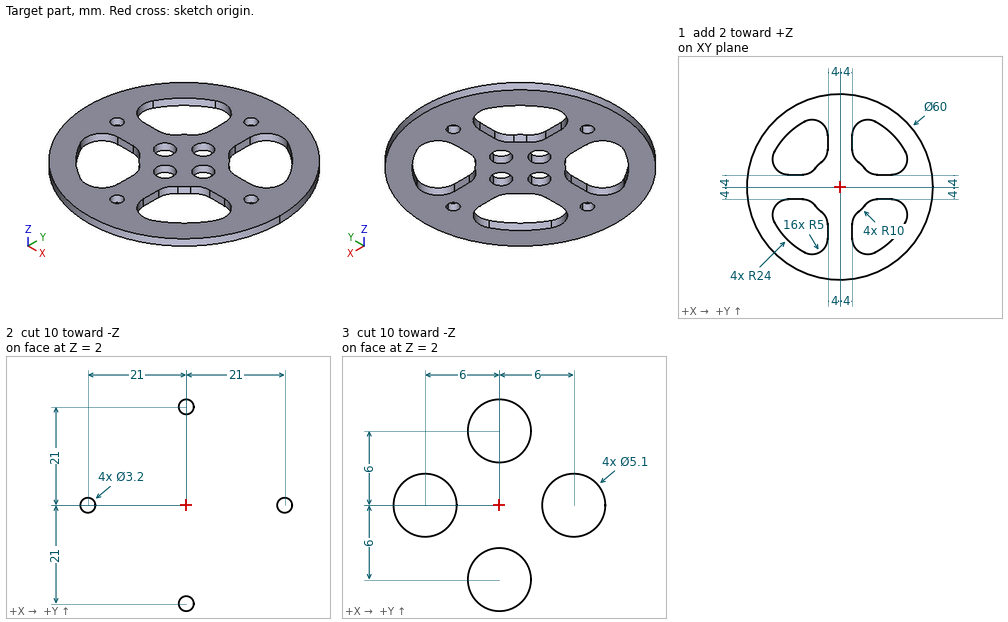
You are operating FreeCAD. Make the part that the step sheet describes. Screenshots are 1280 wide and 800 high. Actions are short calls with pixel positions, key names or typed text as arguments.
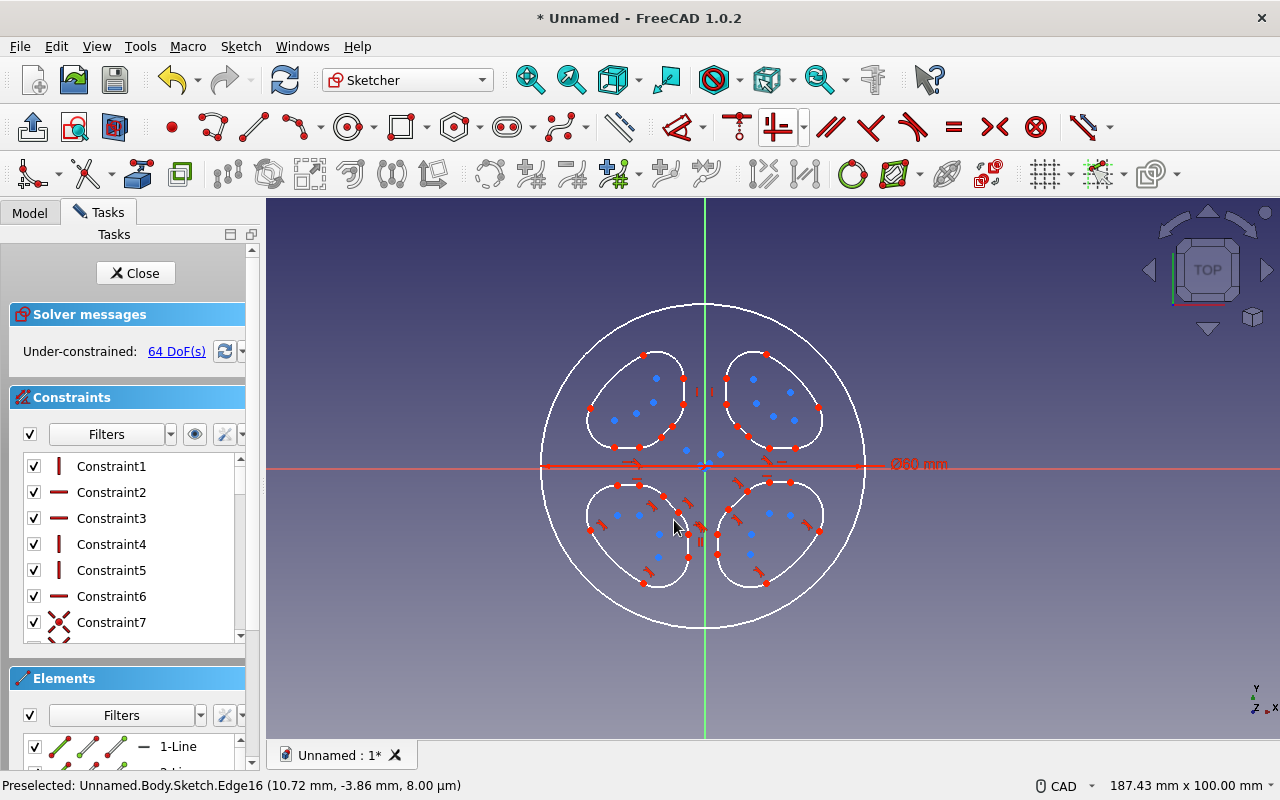
scroll(684, 387, up, 3)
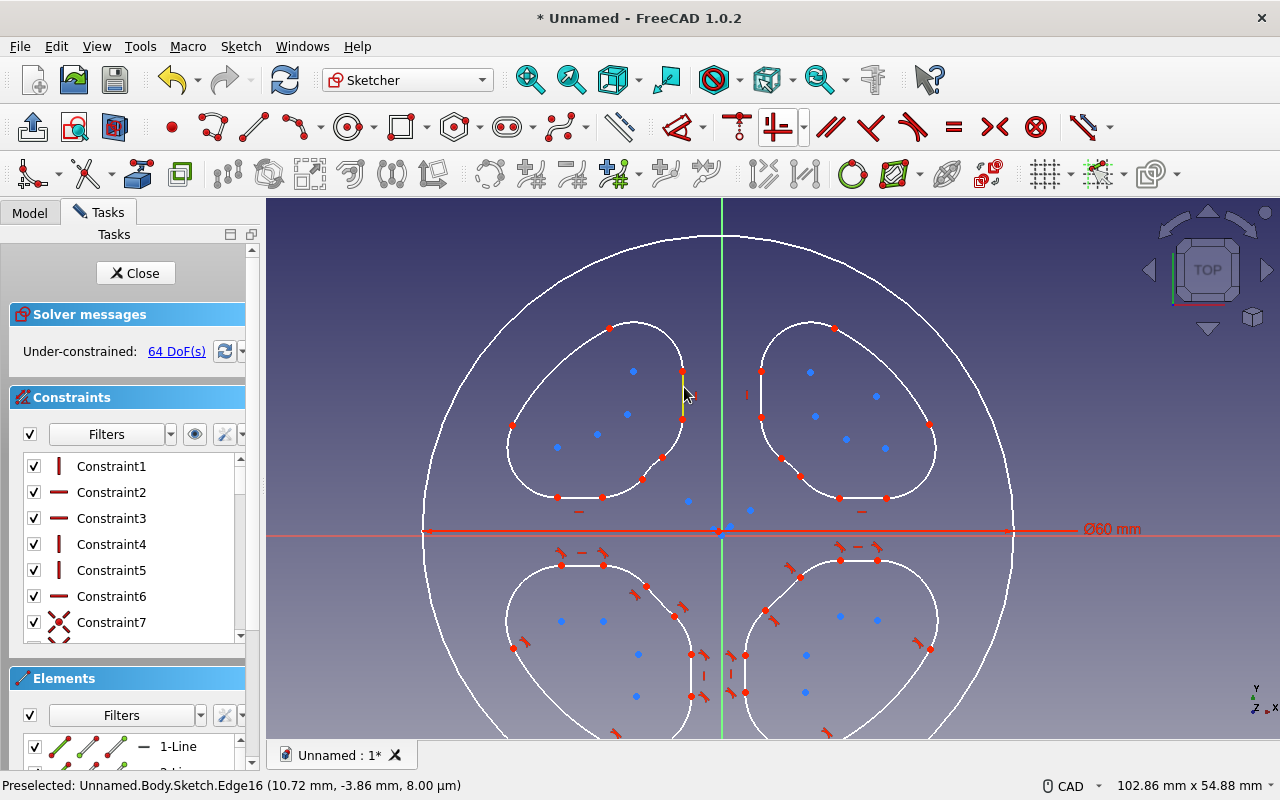
click(683, 386)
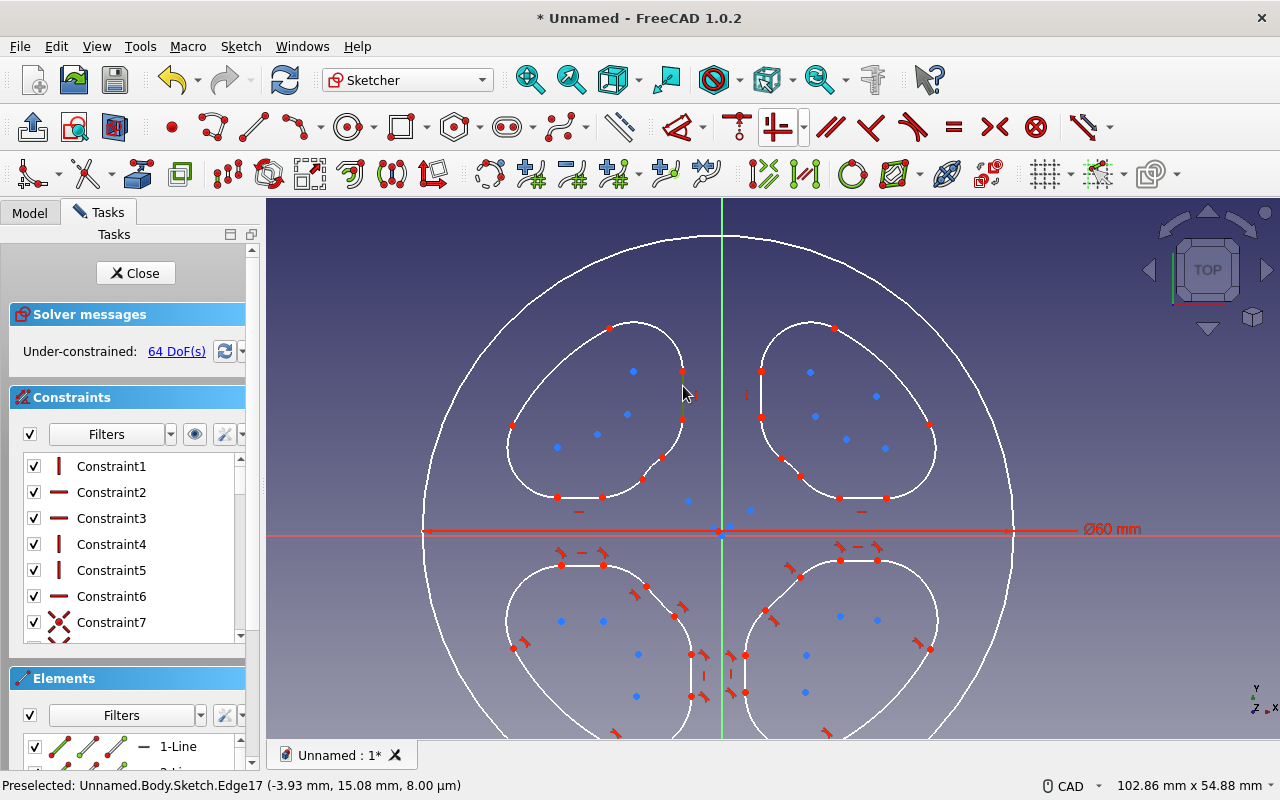
click(672, 448)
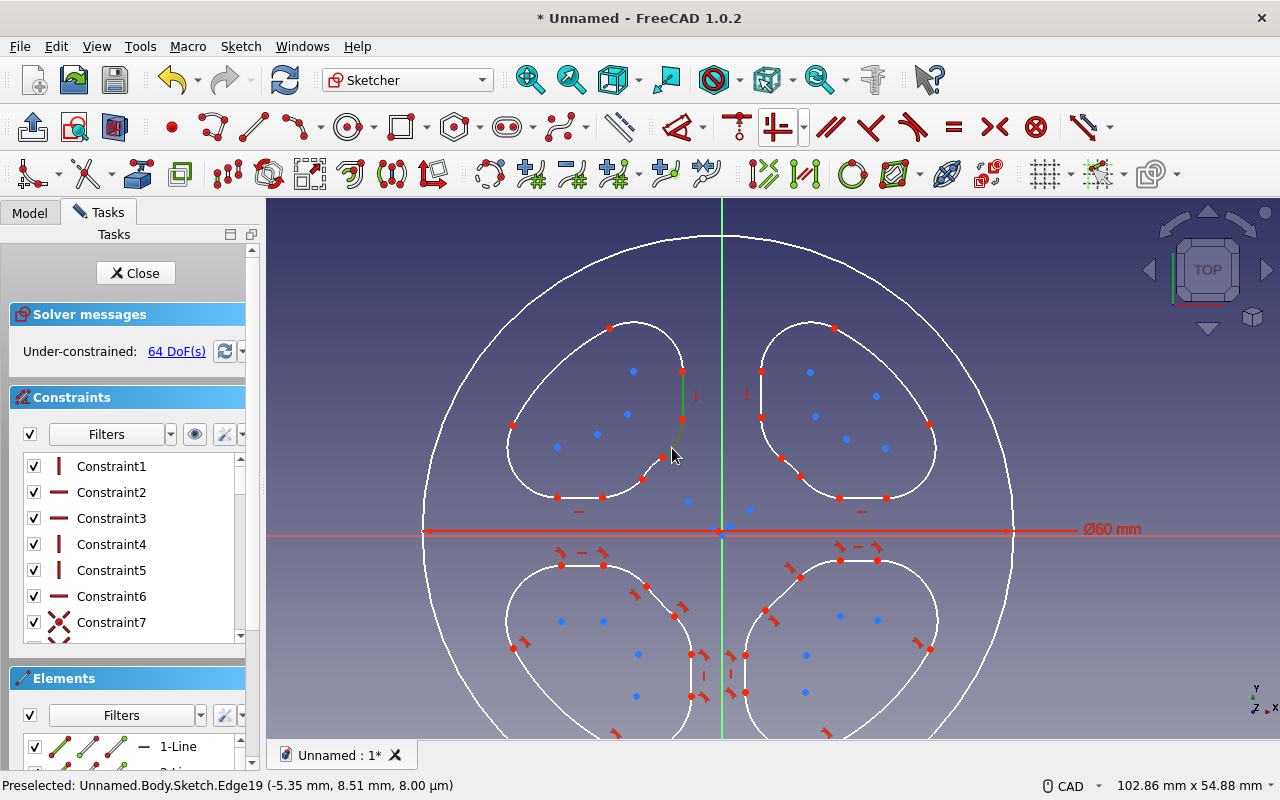
key(t)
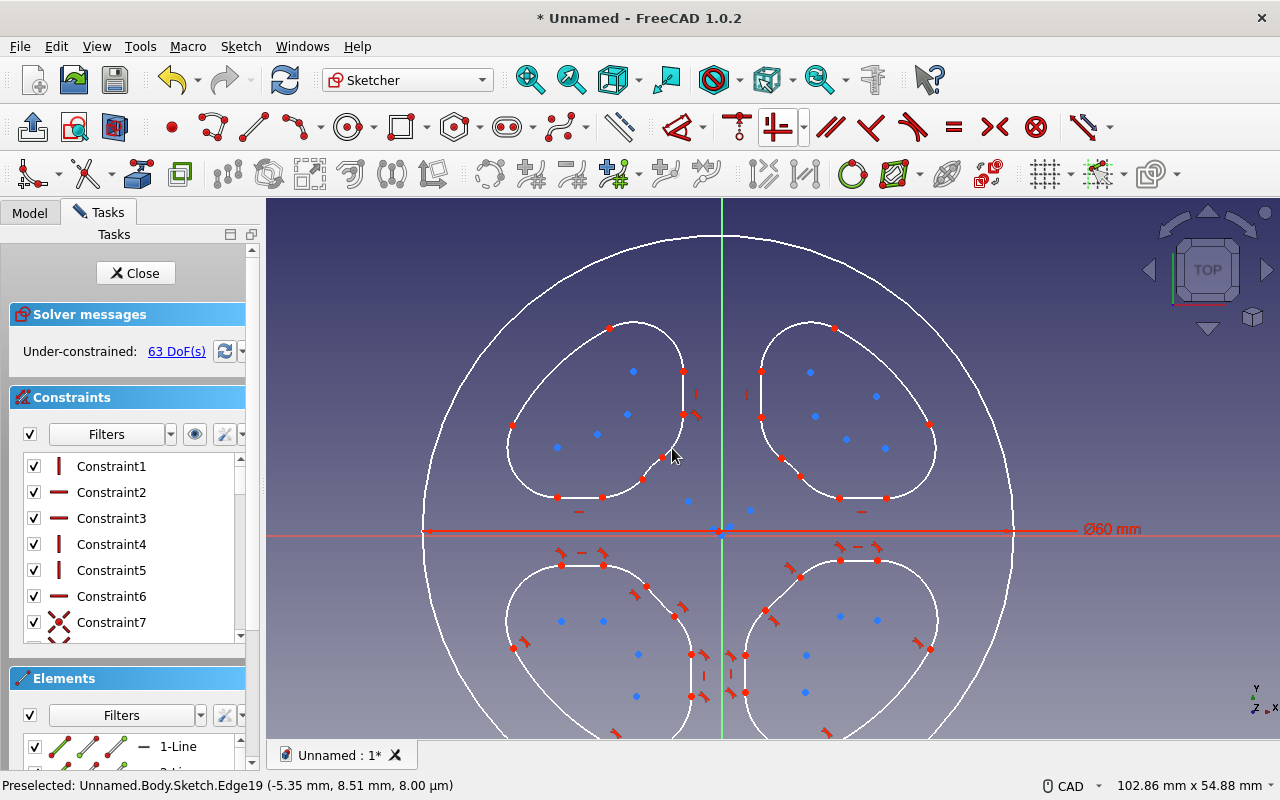
click(683, 385)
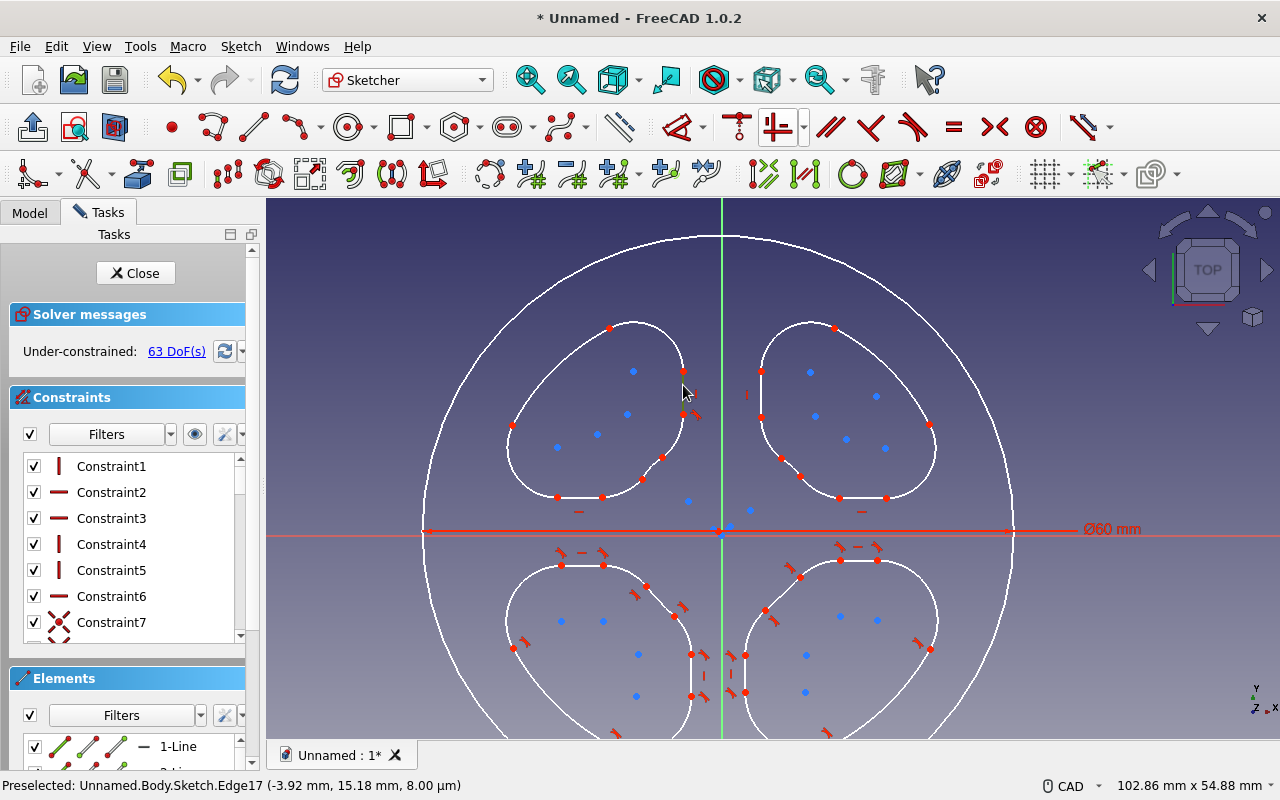
click(674, 343)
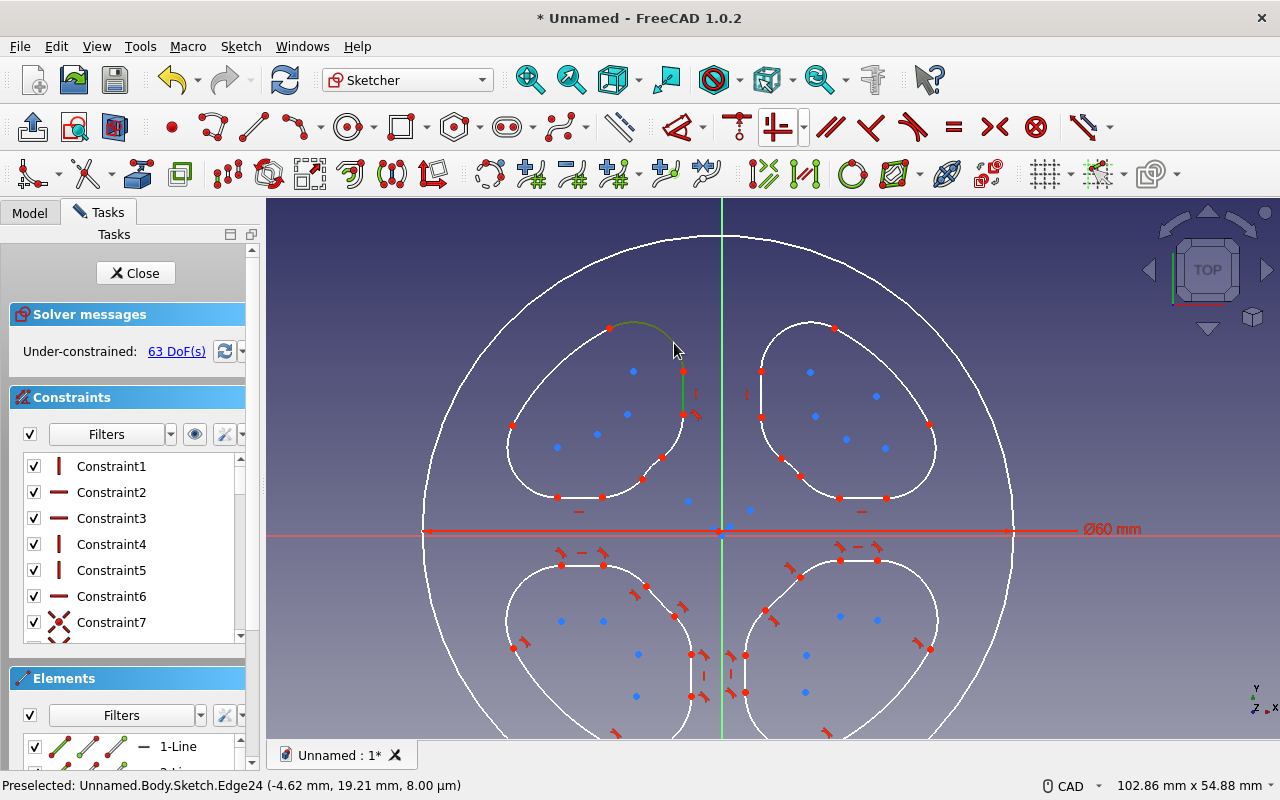
click(913, 128)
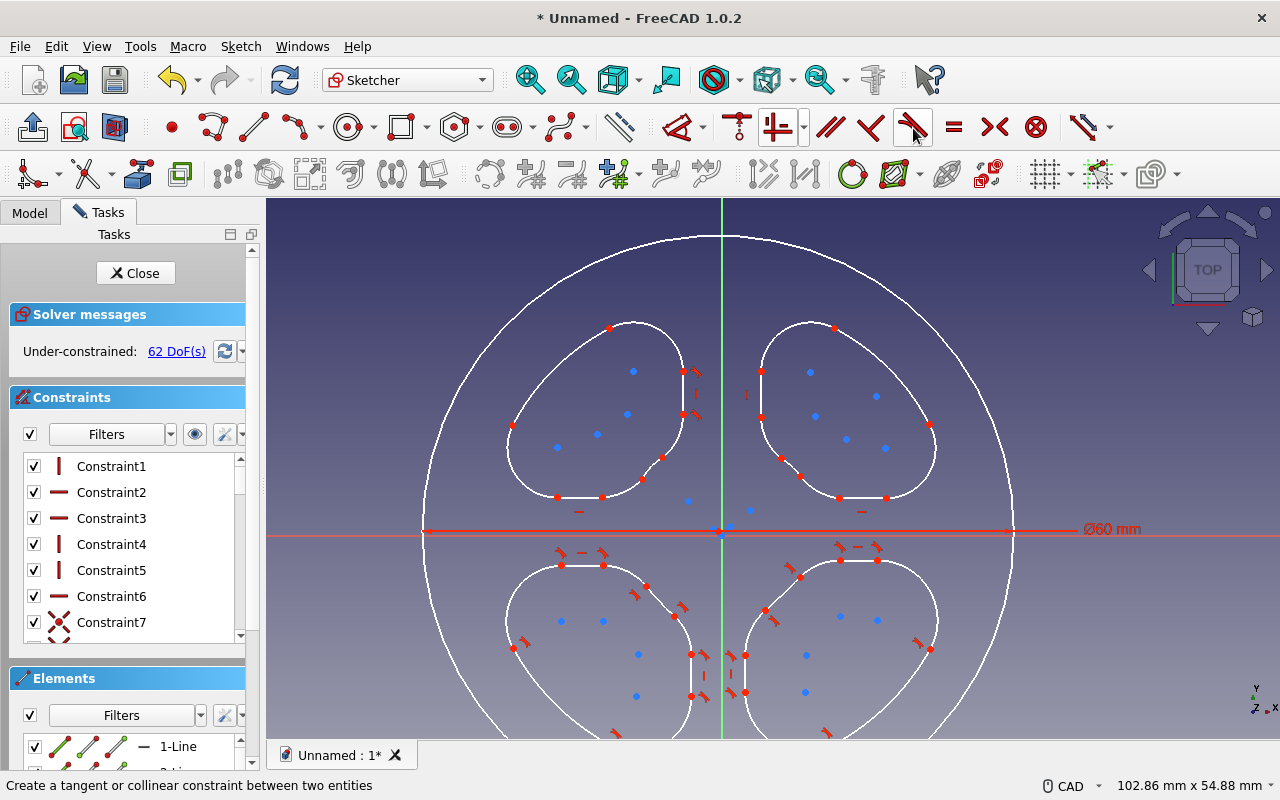
click(589, 498)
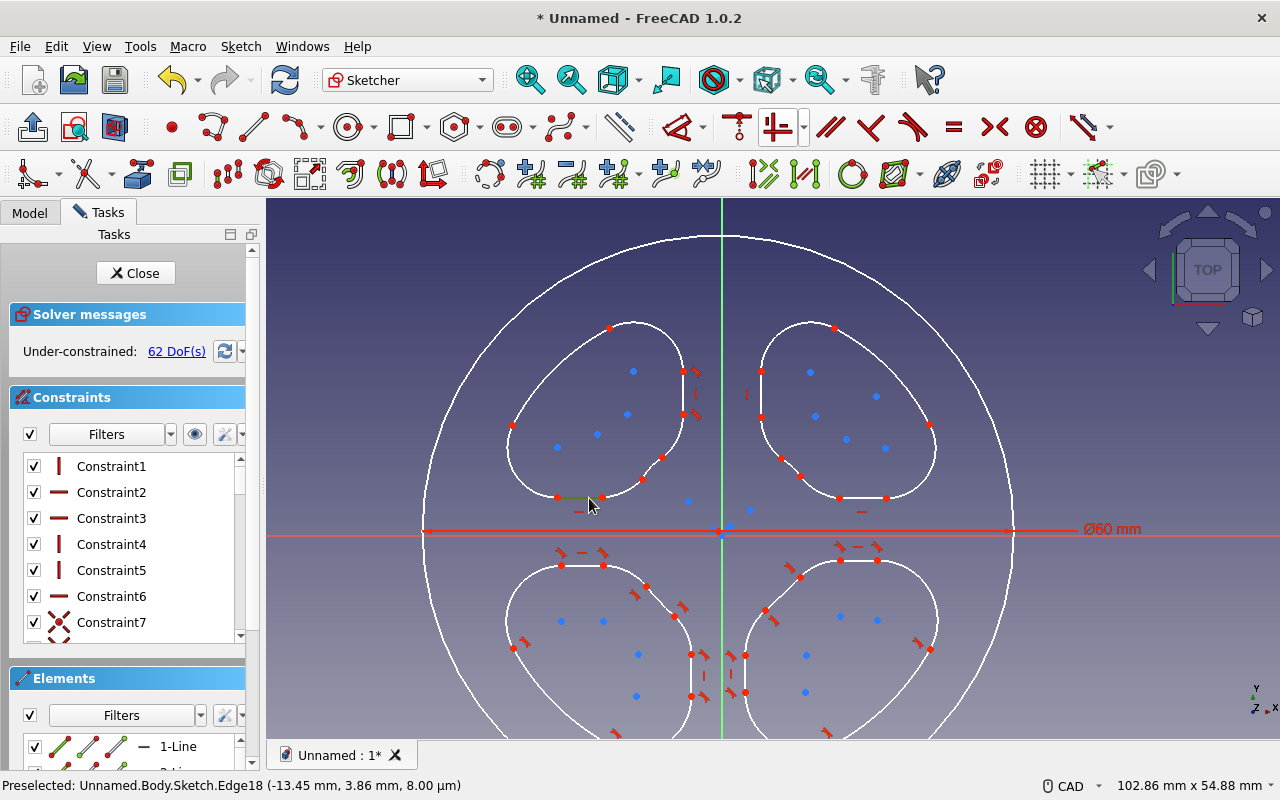
click(616, 495)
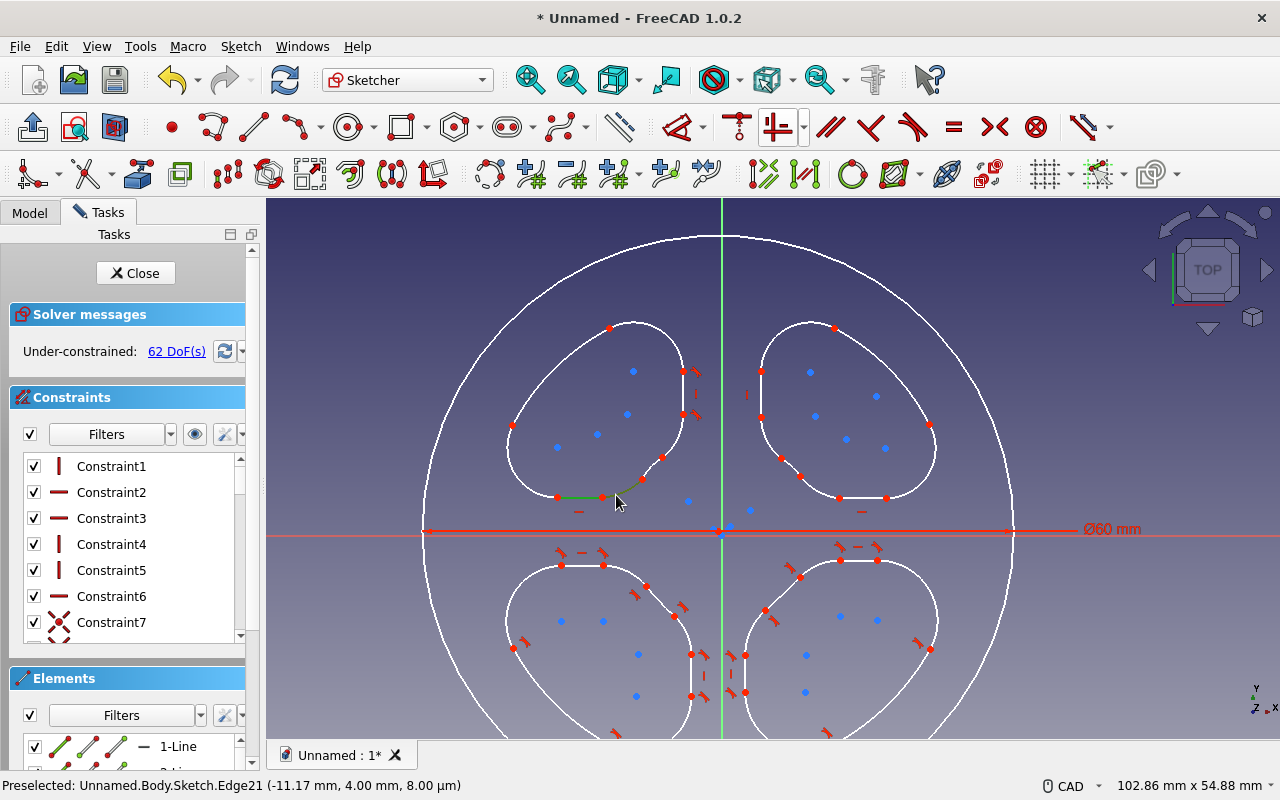
click(913, 128)